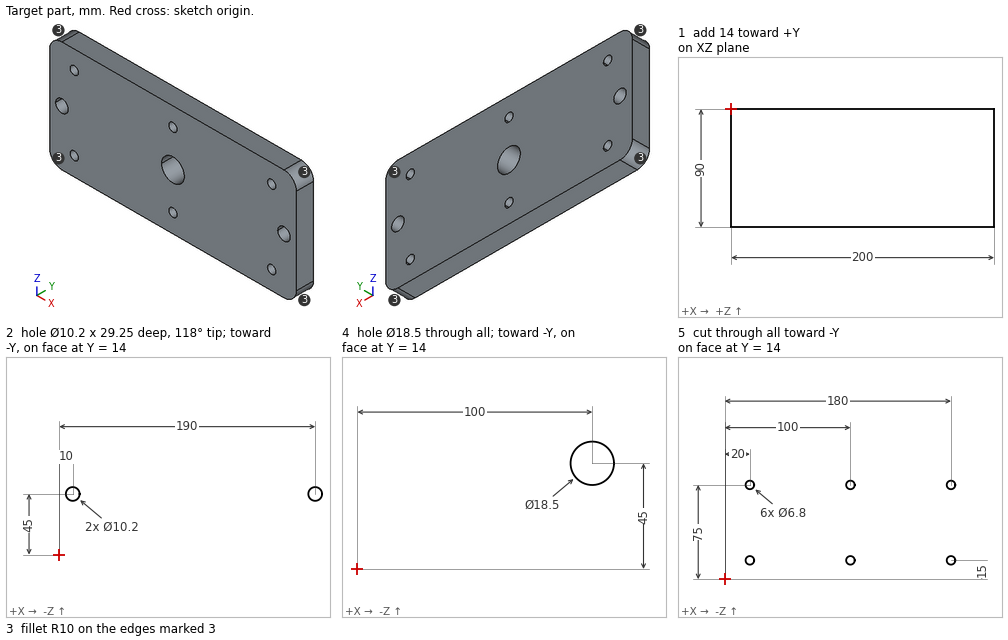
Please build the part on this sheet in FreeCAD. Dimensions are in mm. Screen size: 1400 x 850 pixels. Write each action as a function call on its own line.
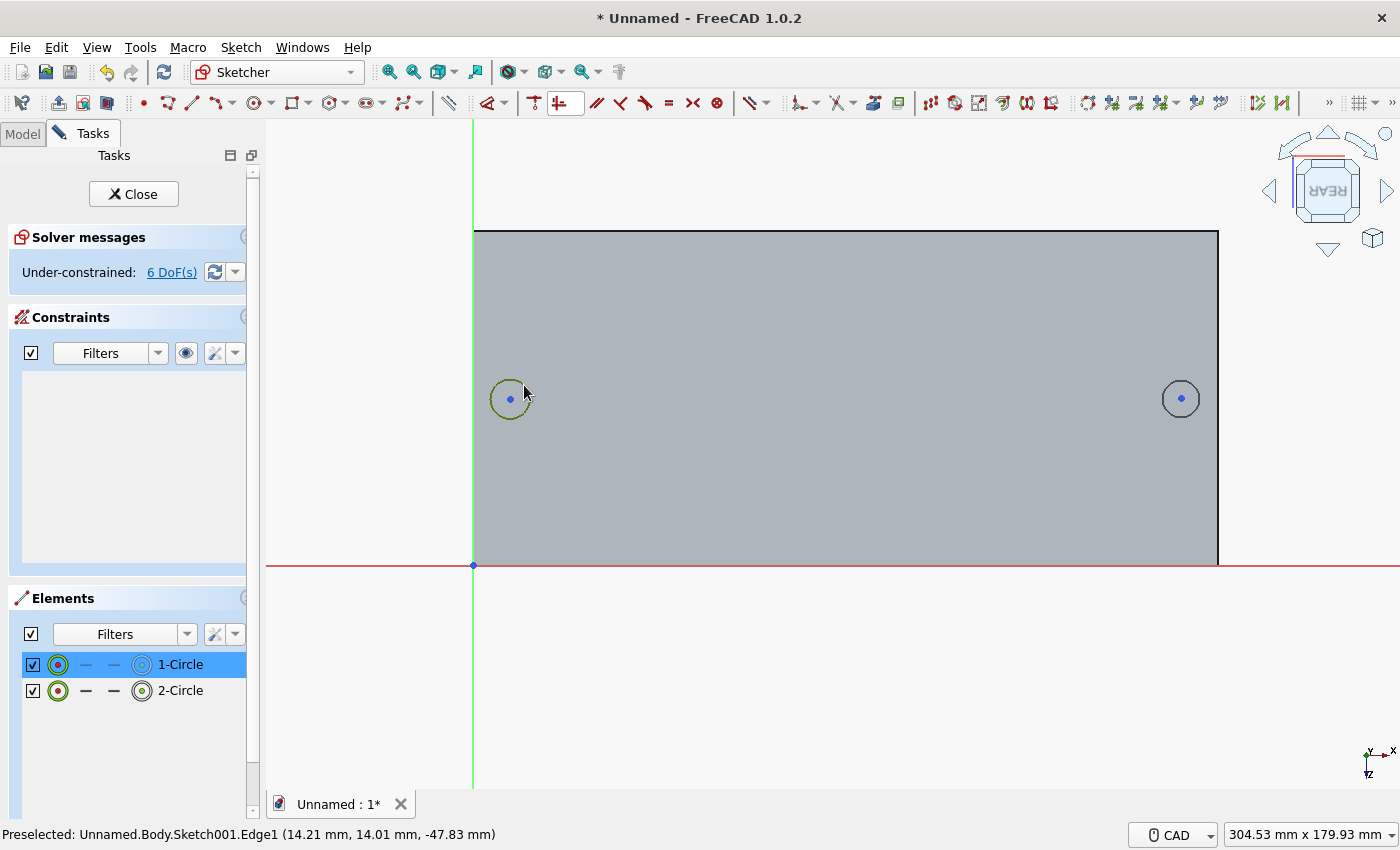
click(1194, 386)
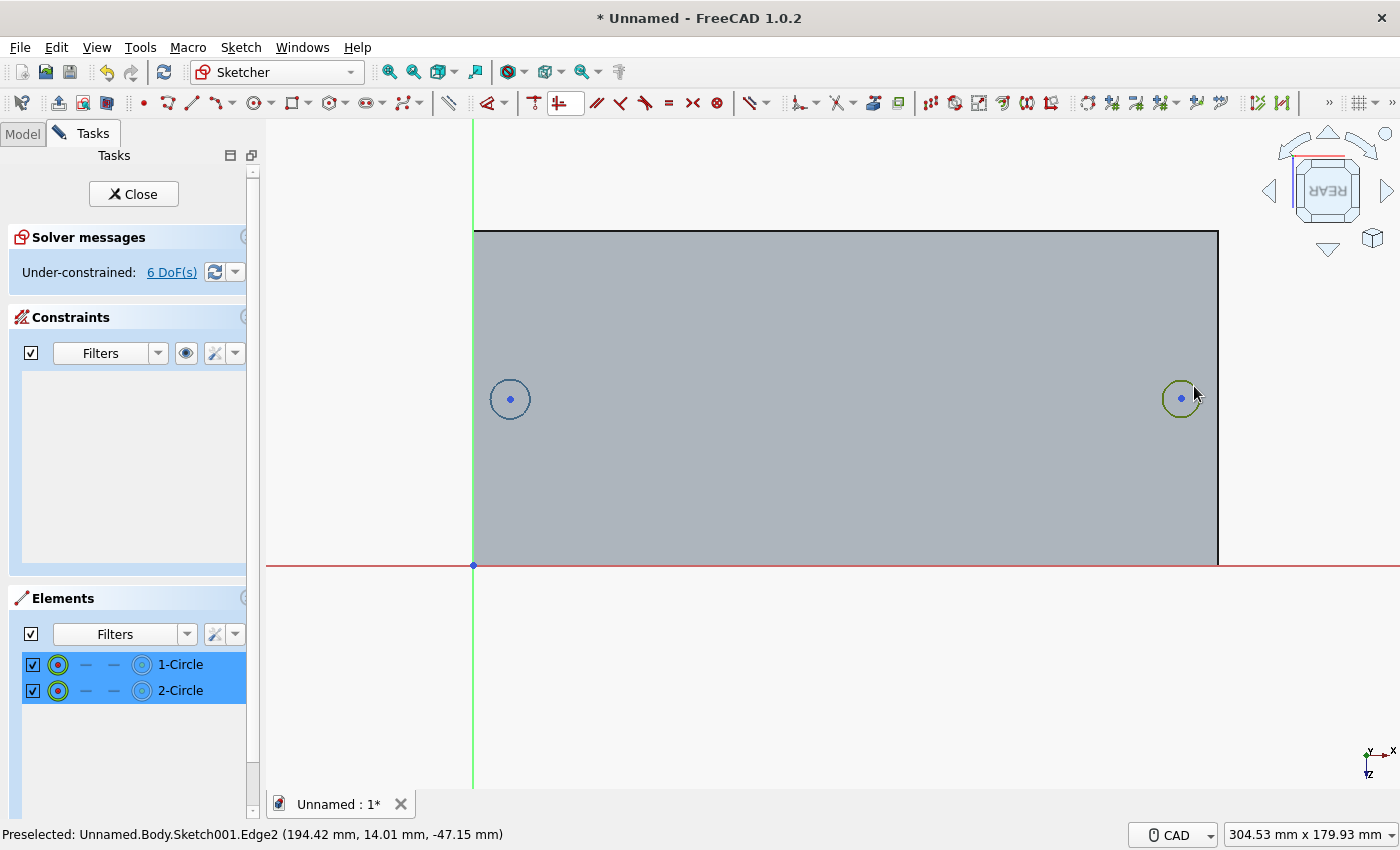
click(670, 104)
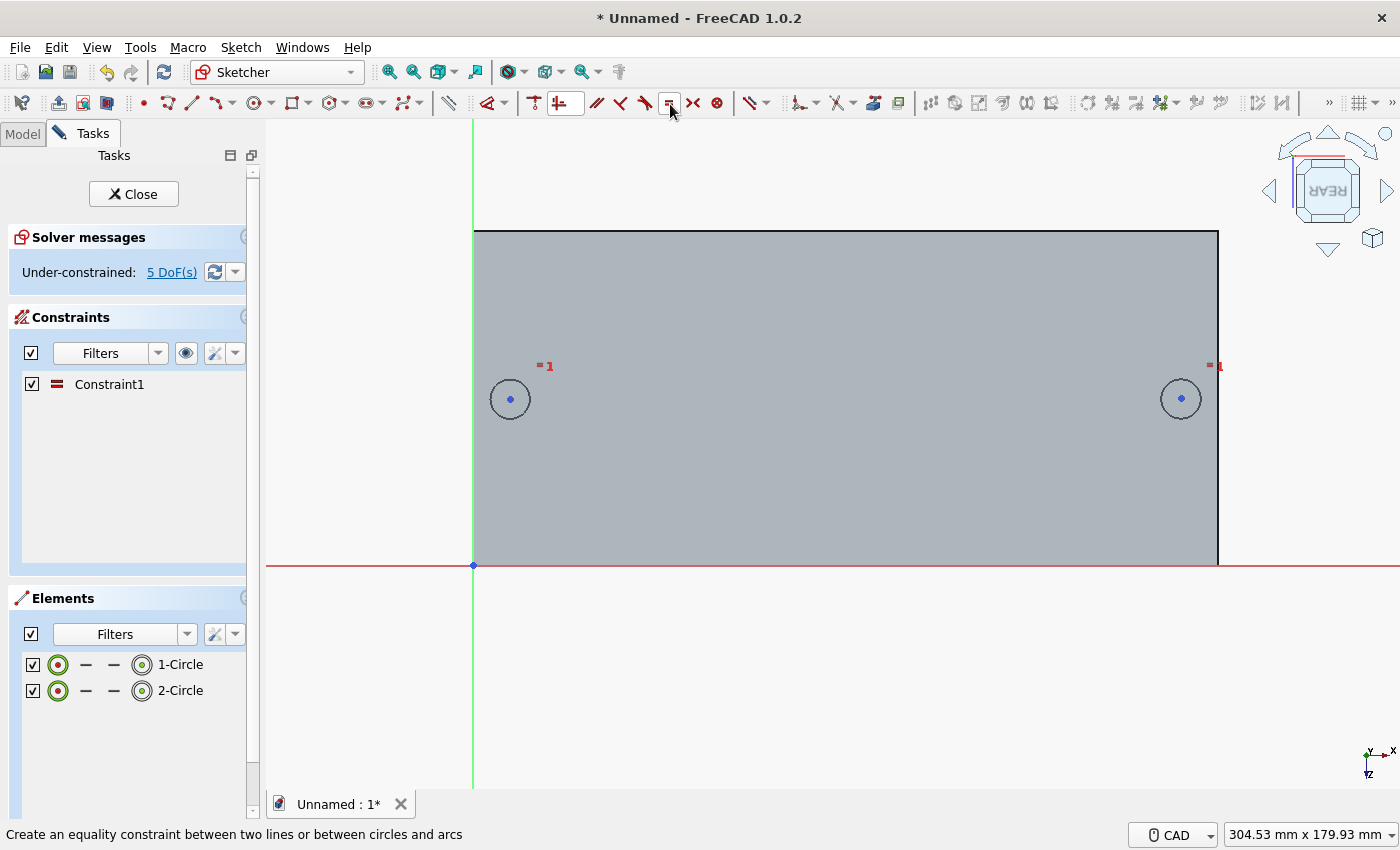
click(510, 399)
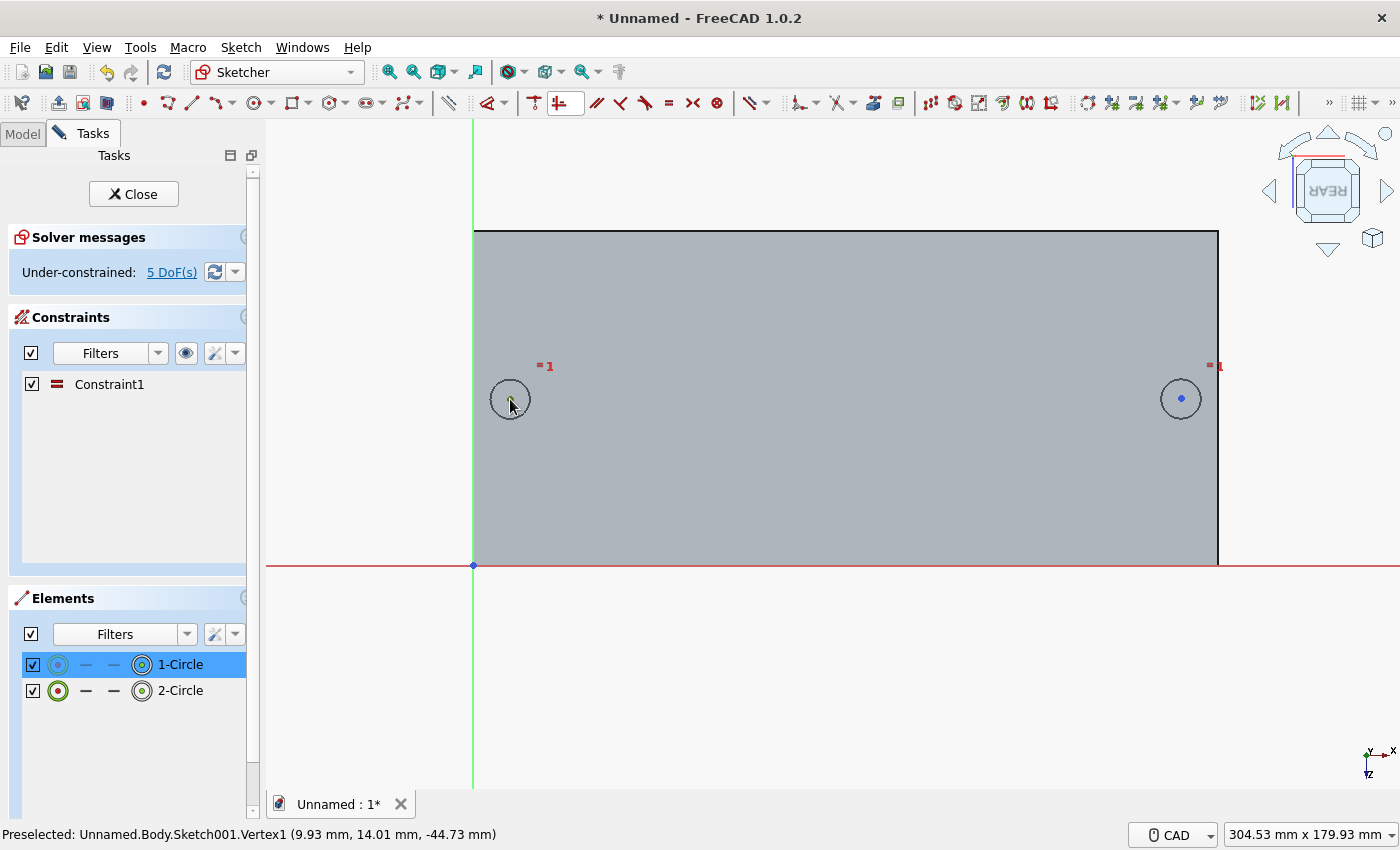
click(1181, 399)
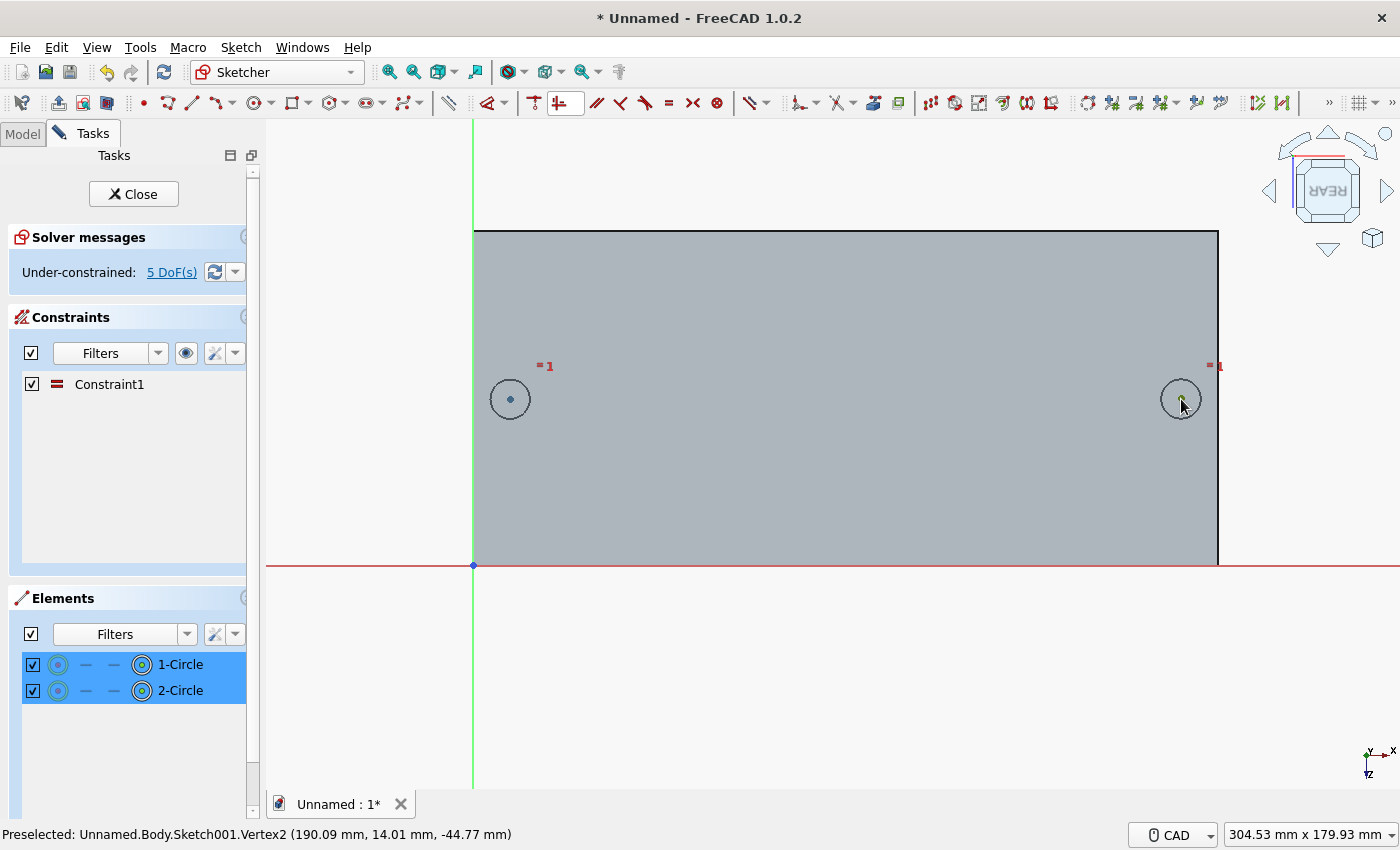
click(578, 104)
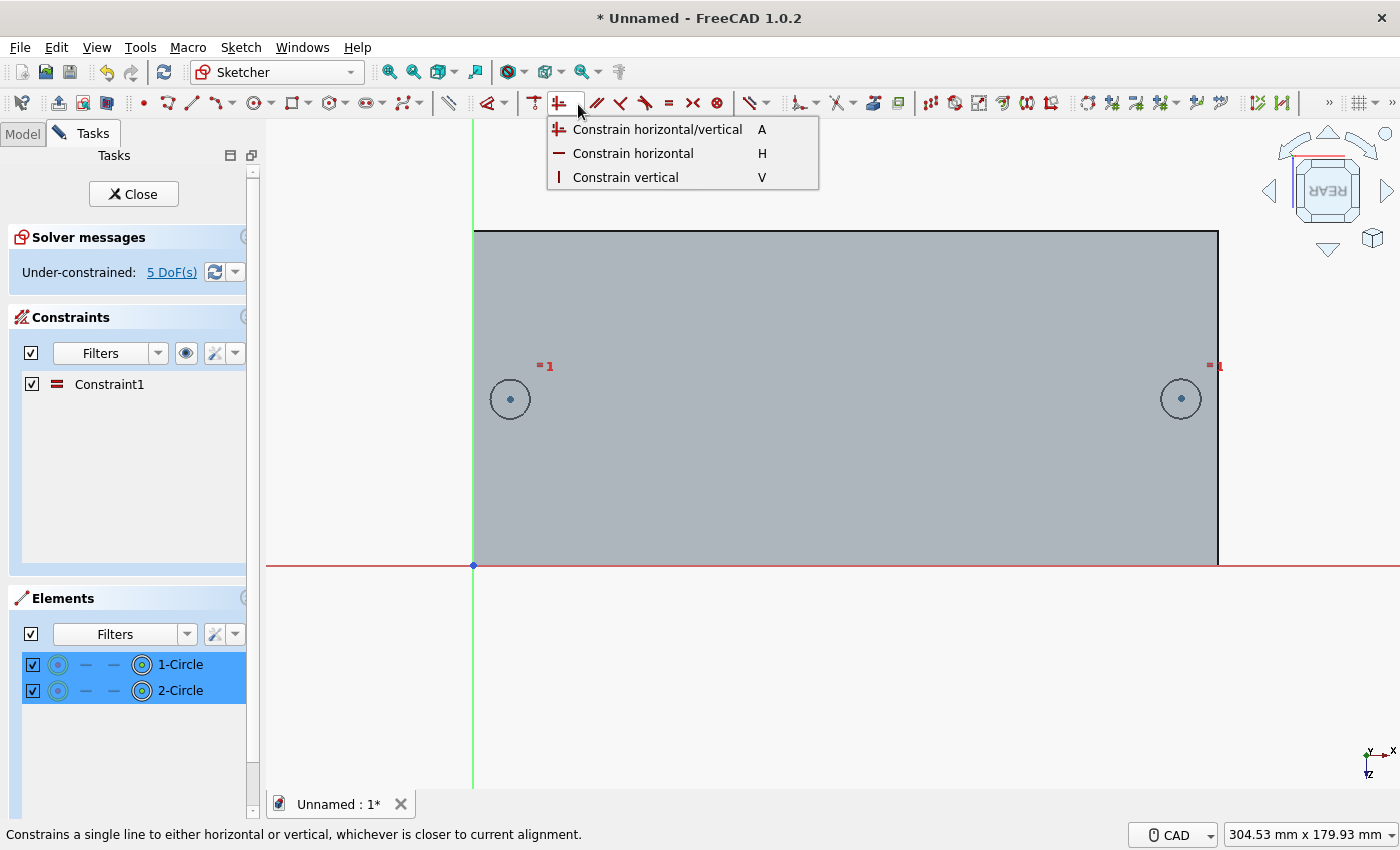
click(683, 153)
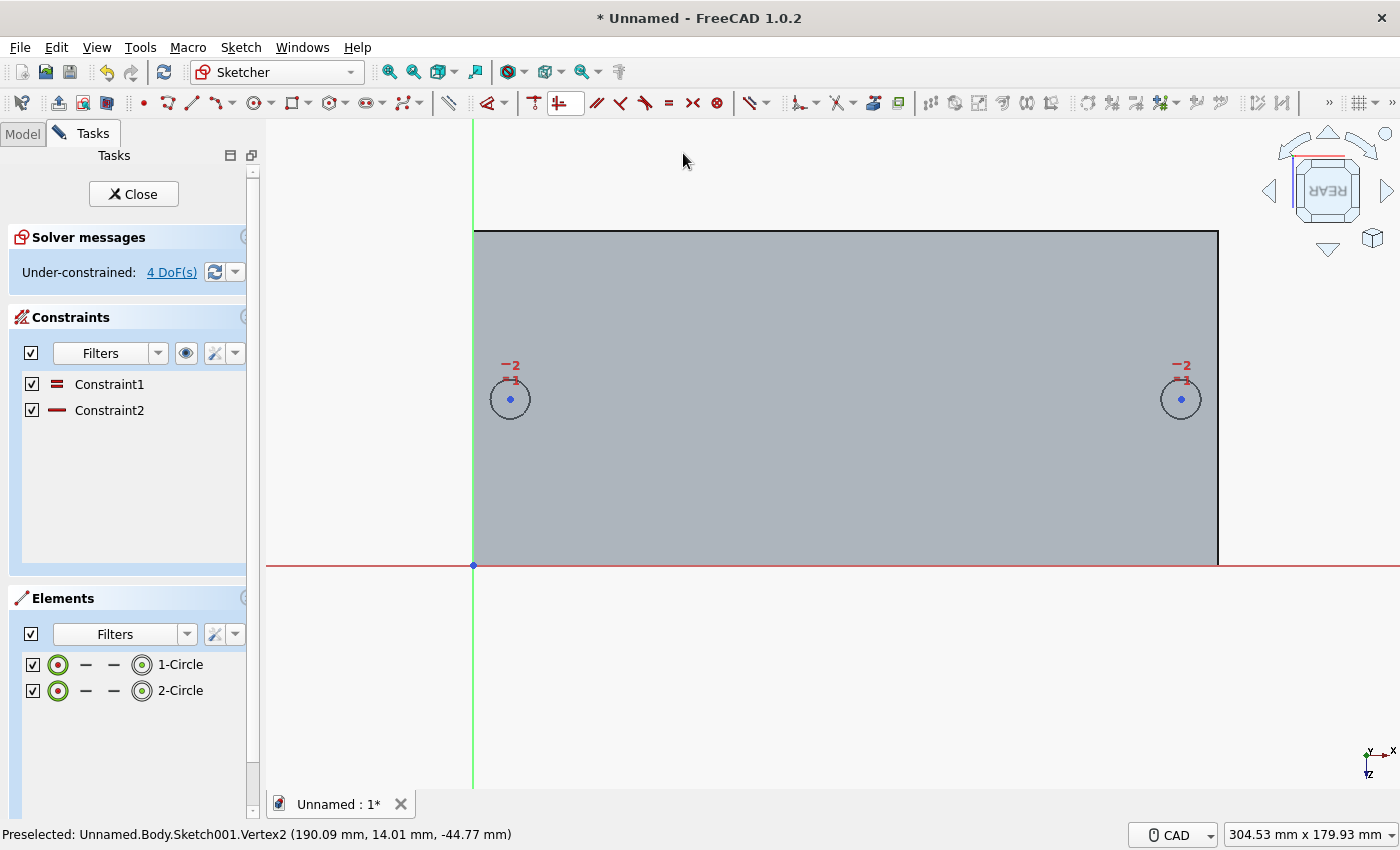
click(488, 104)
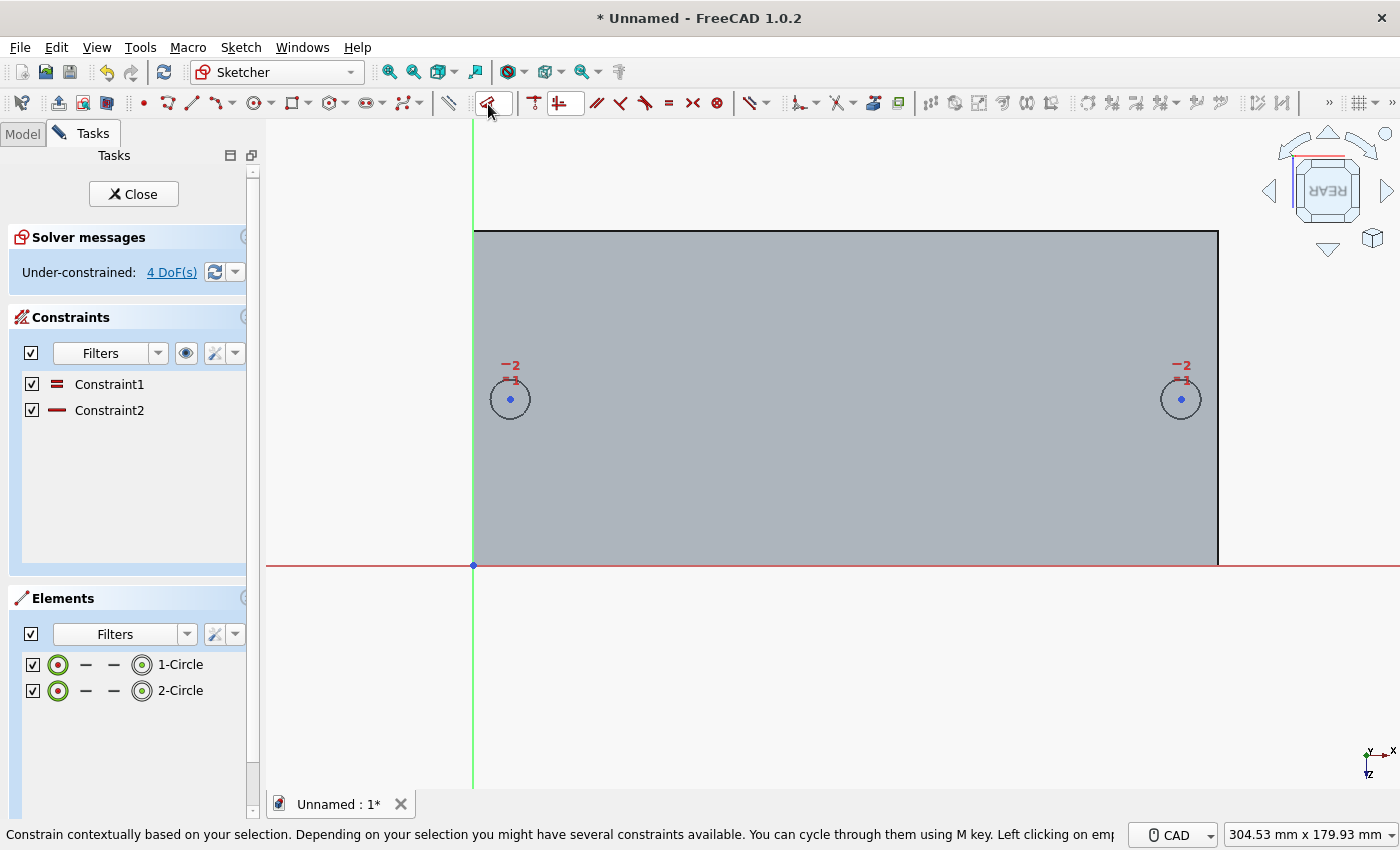
click(524, 385)
click(546, 362)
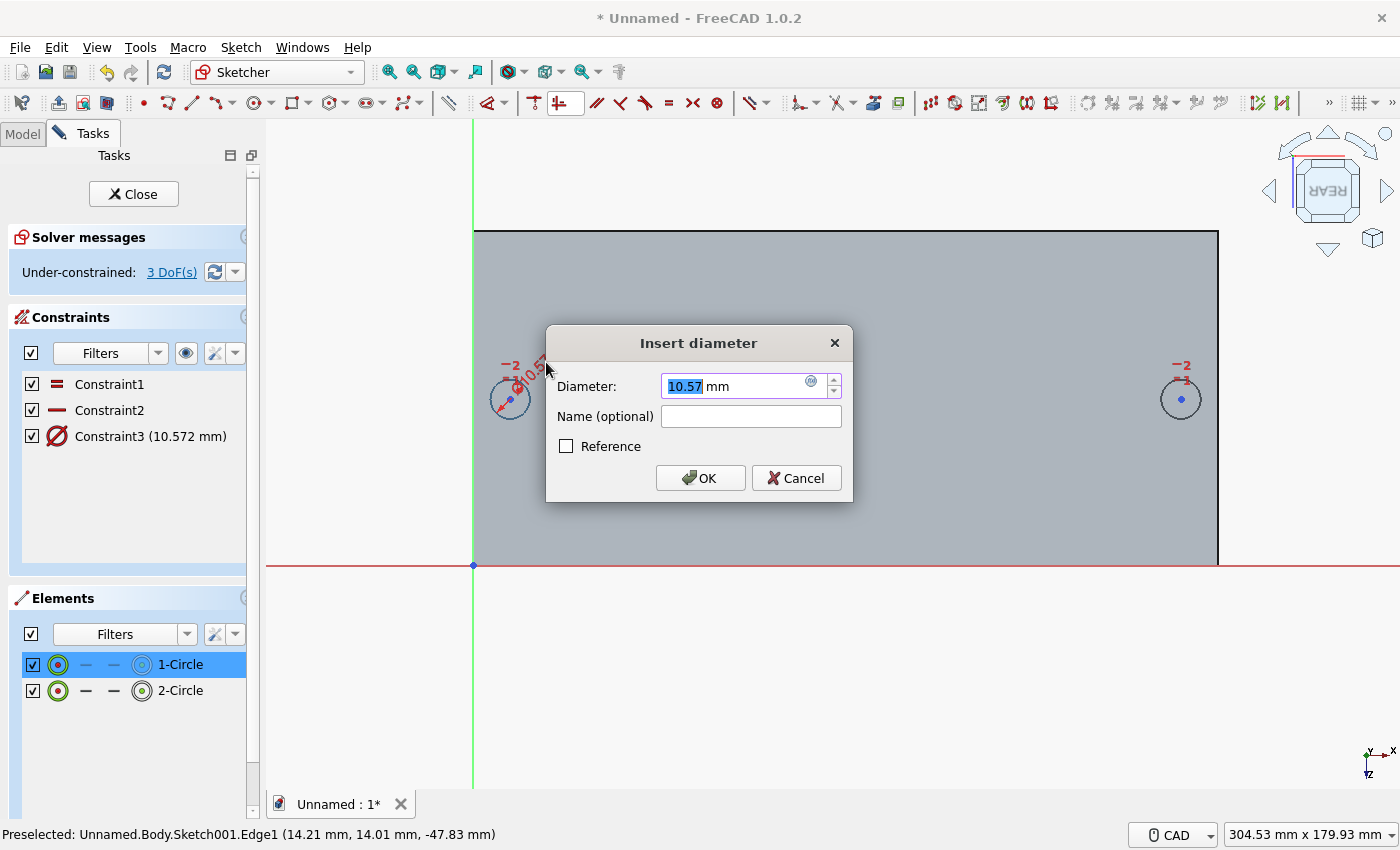
text(10.2)
key(Return)